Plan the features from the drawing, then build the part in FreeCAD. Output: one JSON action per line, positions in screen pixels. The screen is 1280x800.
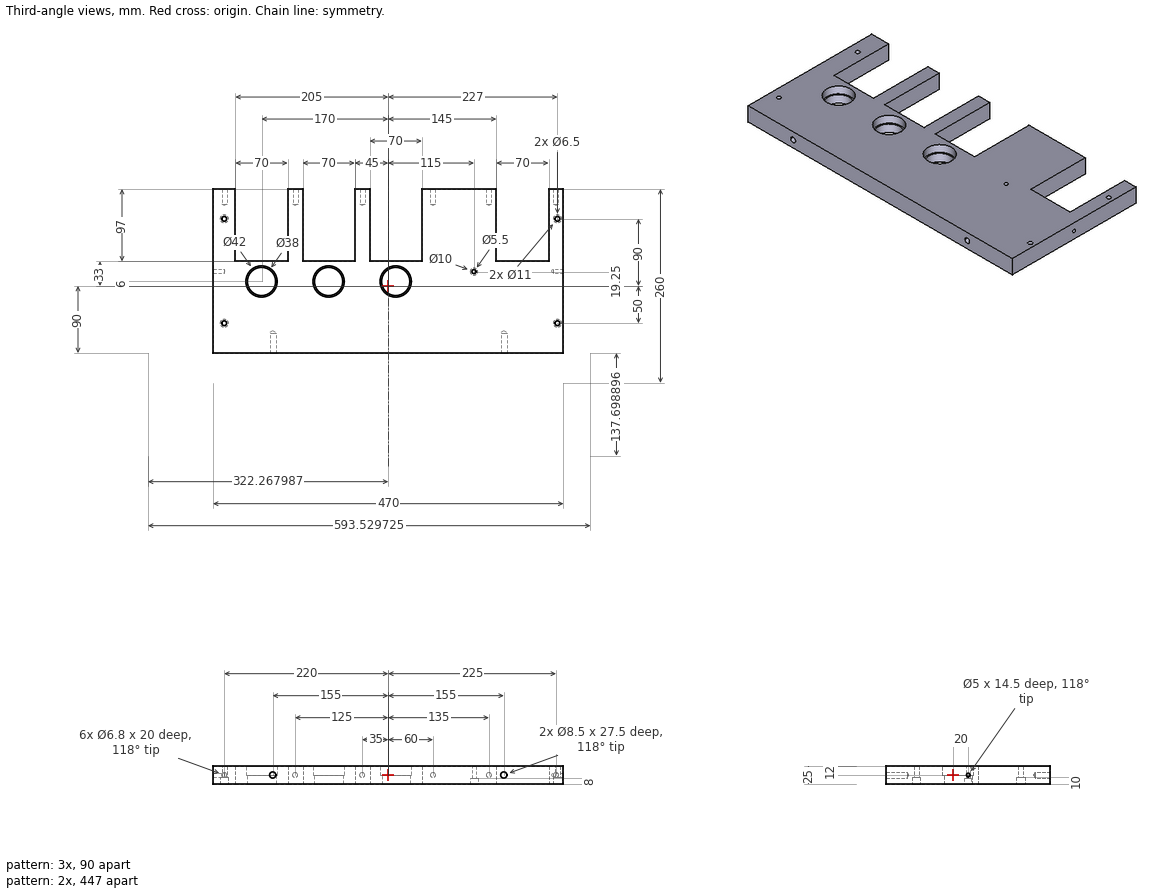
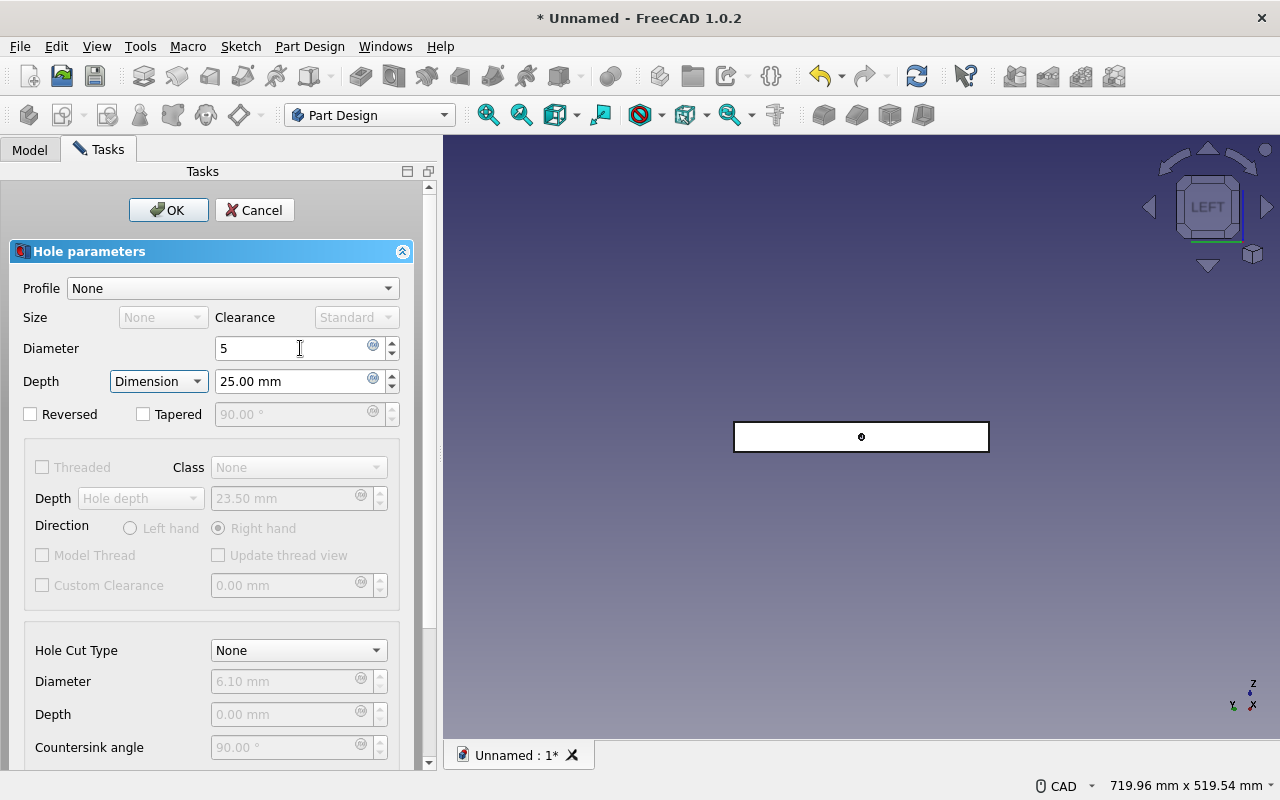
{"action": "triple_click", "coordinate": [300, 382]}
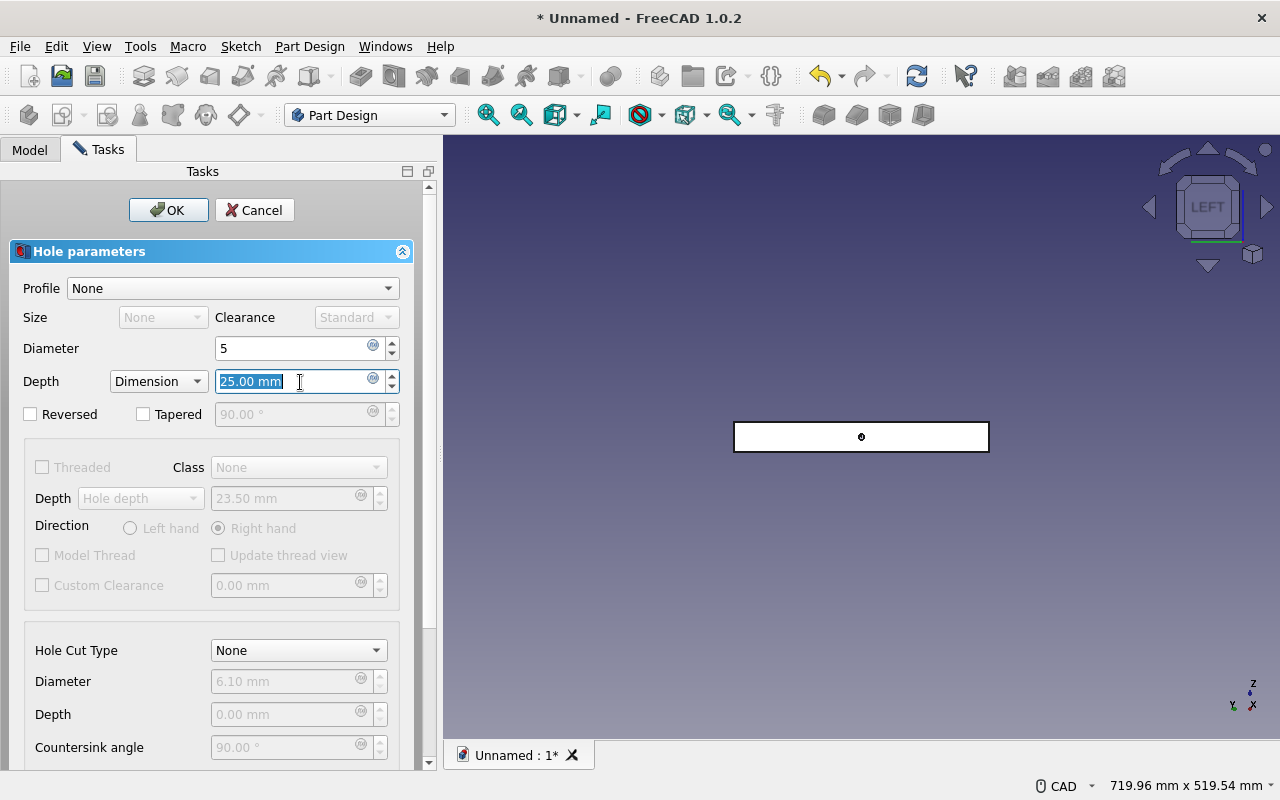
{"action": "type", "text": "14.5"}
{"action": "key", "text": "Tab"}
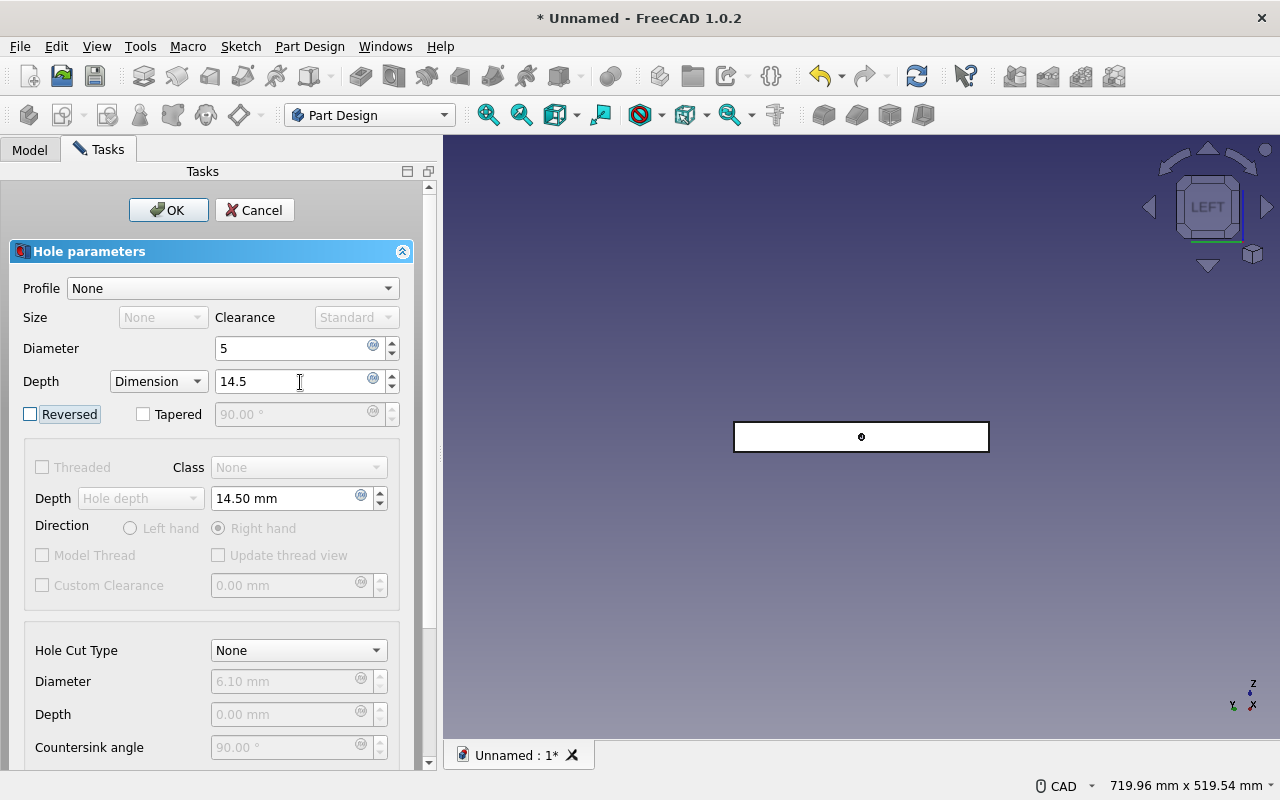
{"action": "left_click", "coordinate": [169, 210]}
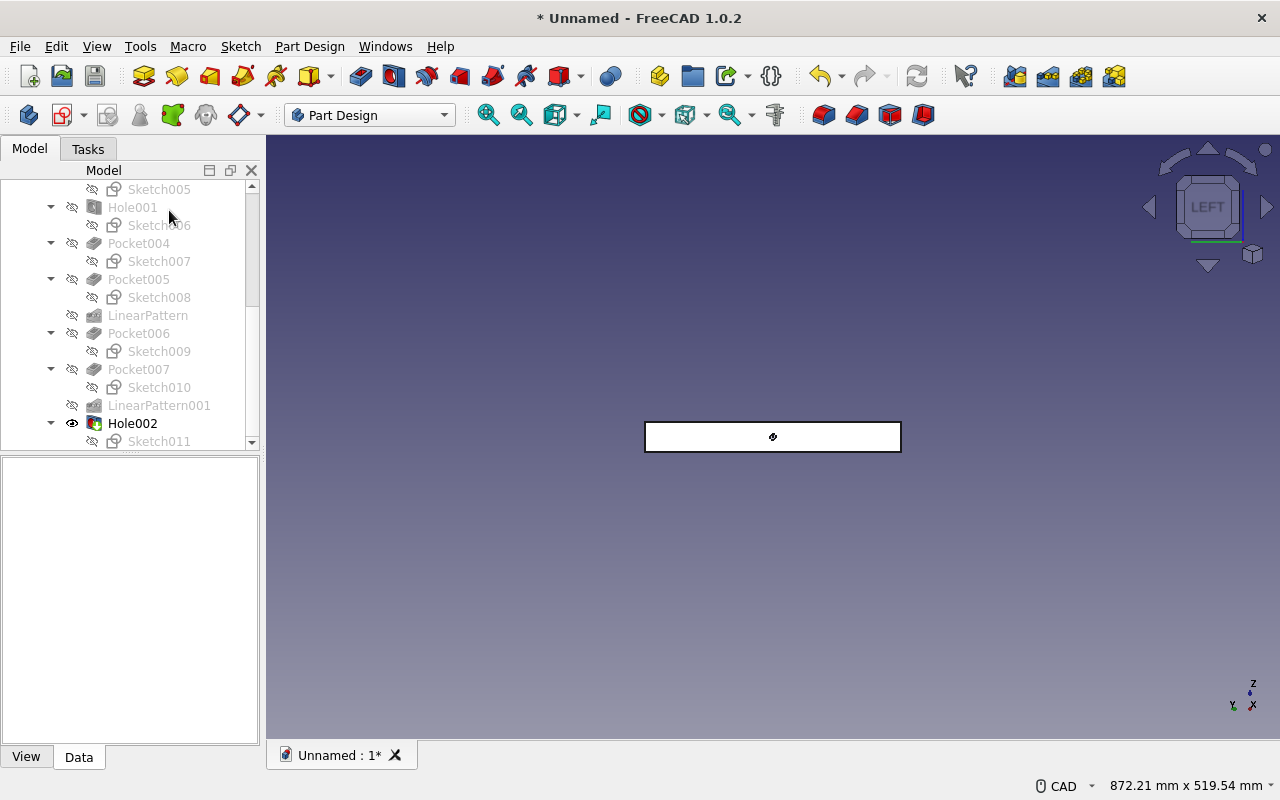
{"action": "left_click", "coordinate": [489, 116]}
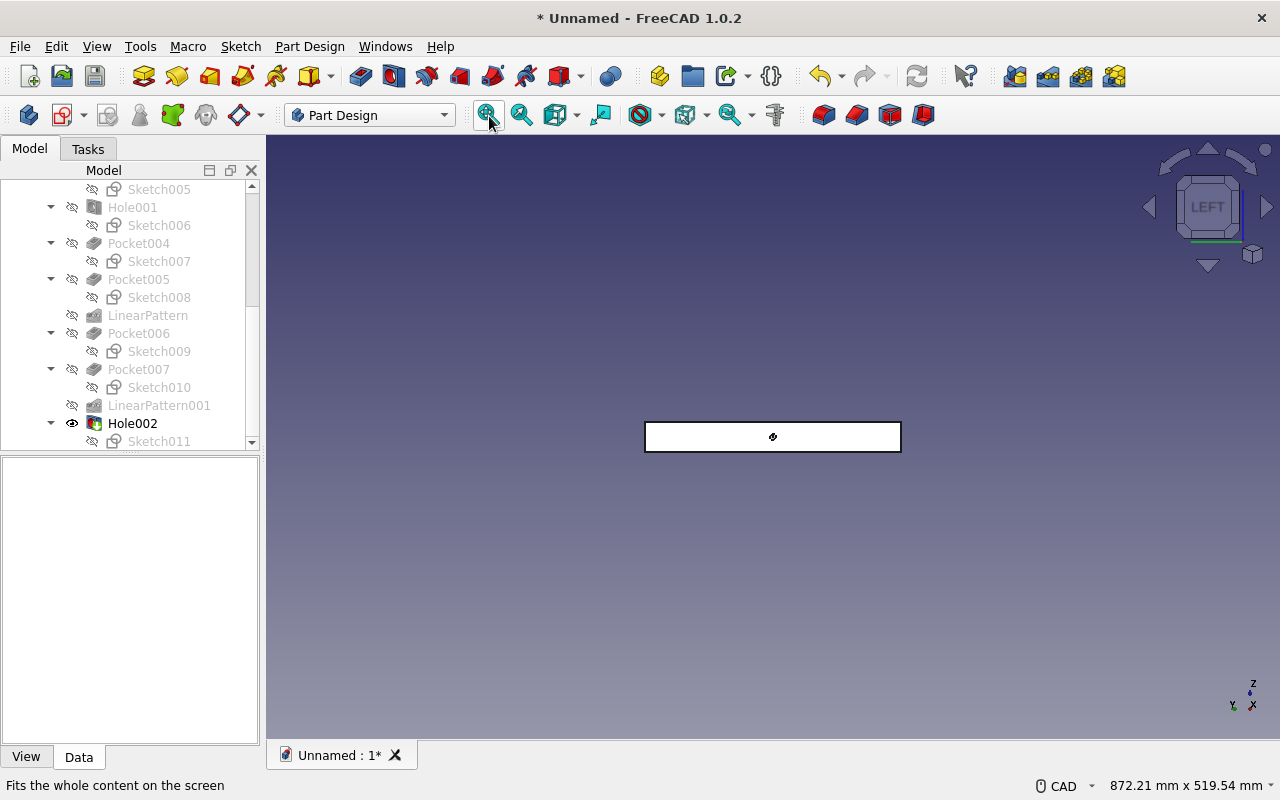
{"action": "key", "text": "0"}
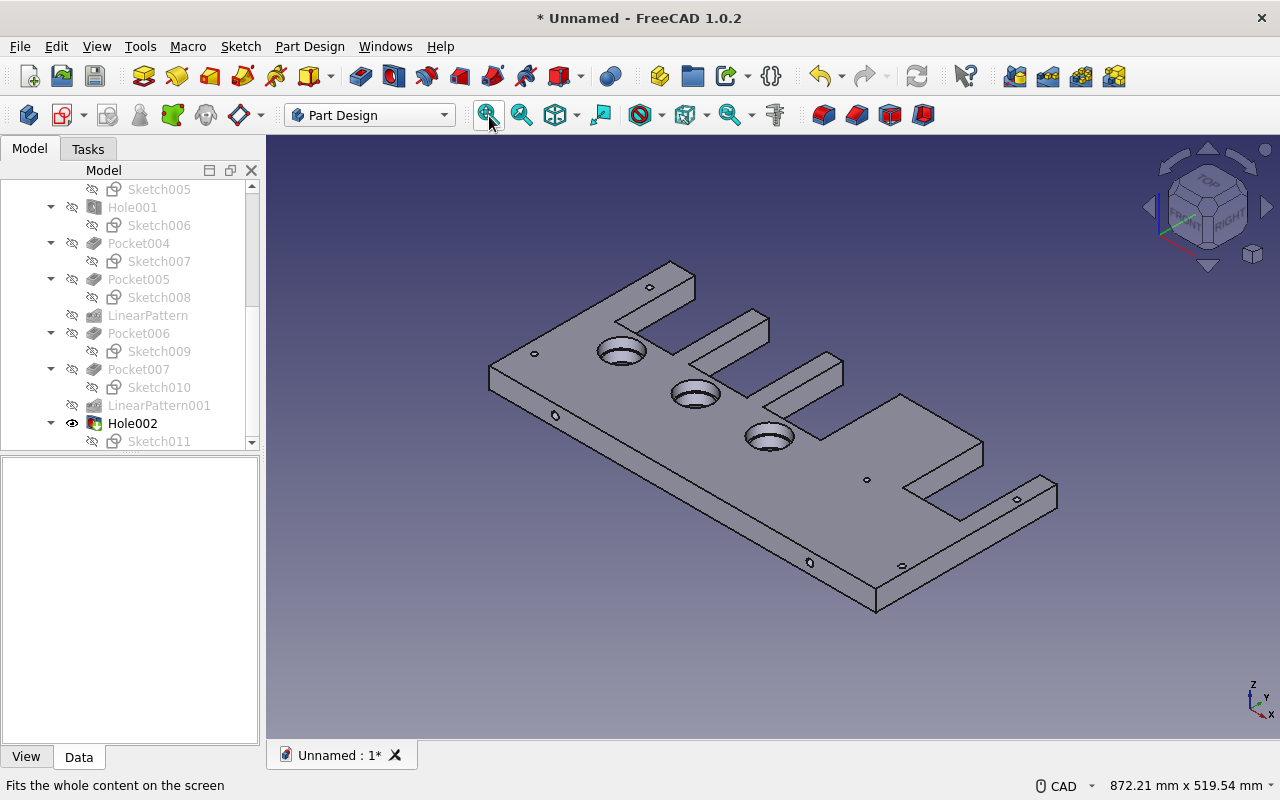
{"action": "left_click", "coordinate": [1044, 503]}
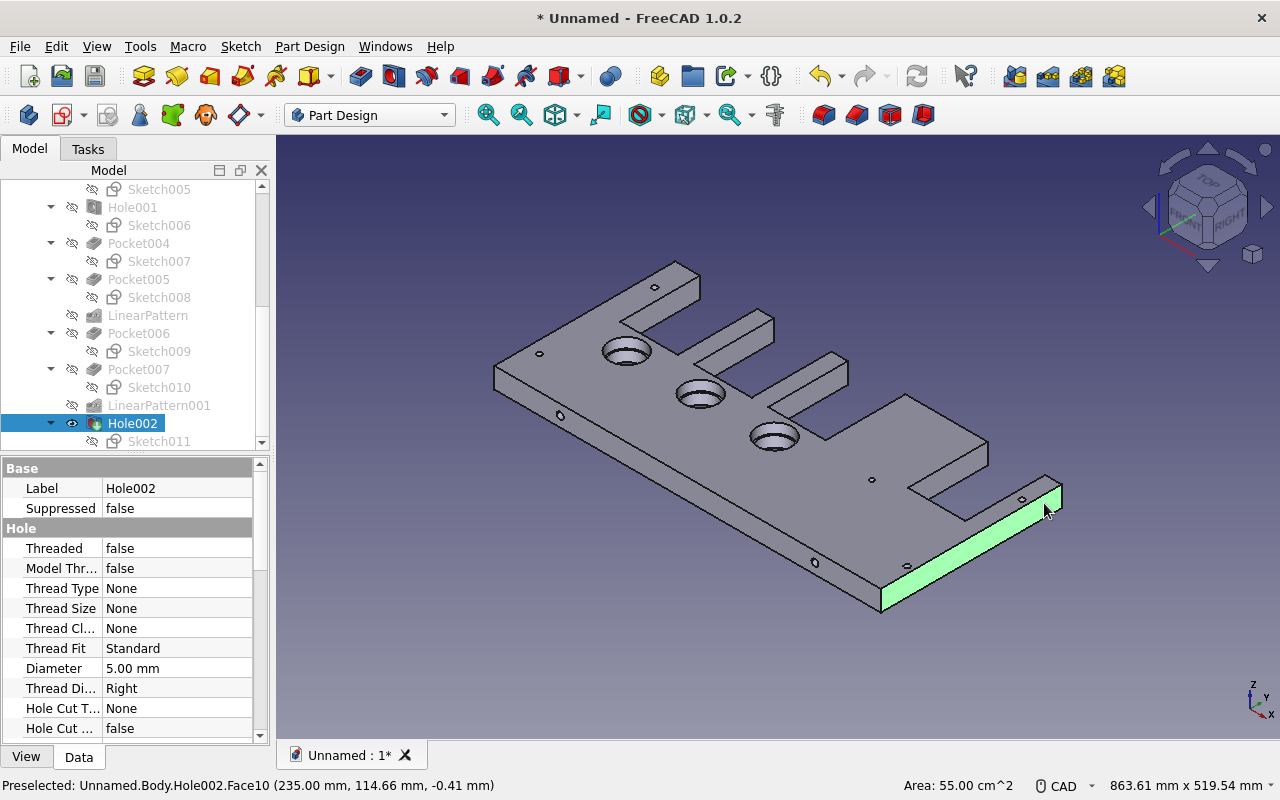
{"action": "left_click", "coordinate": [62, 116]}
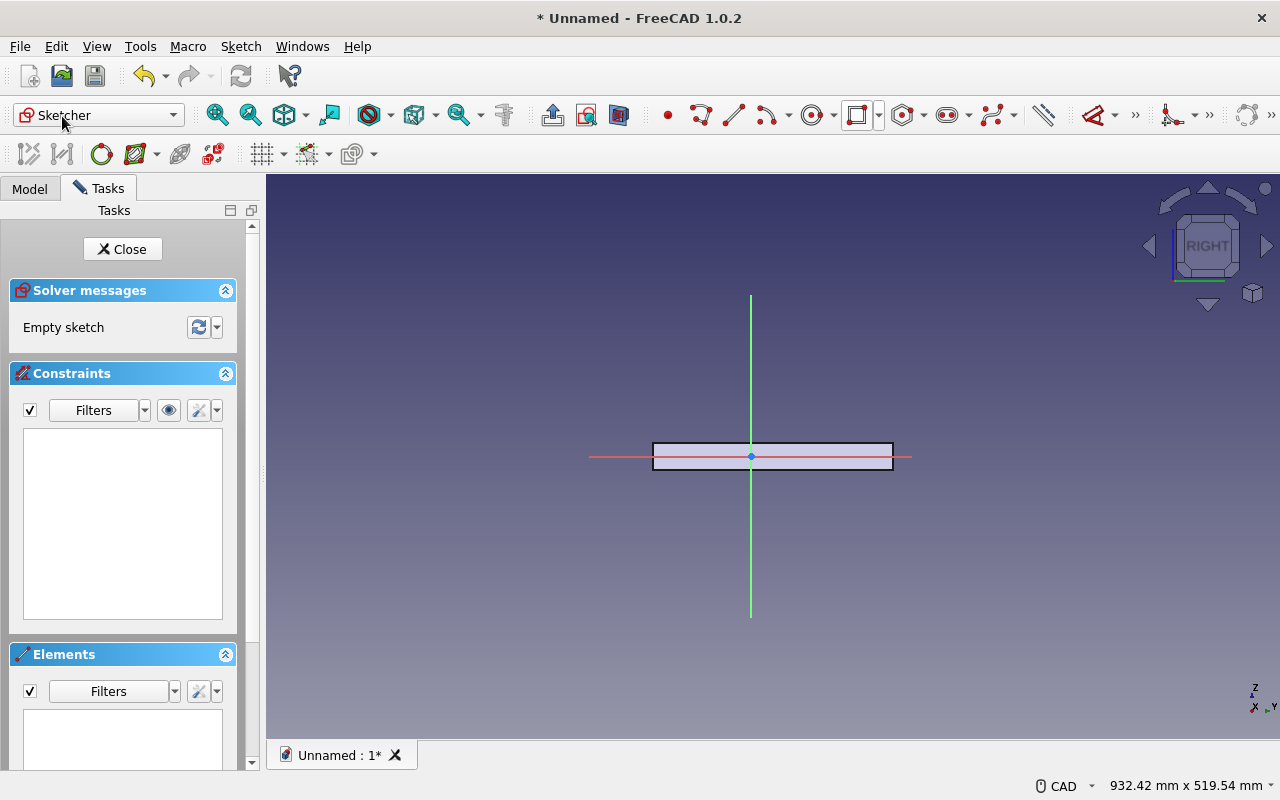
{"action": "scroll", "coordinate": [777, 456], "scroll_direction": "up", "scroll_amount": 15}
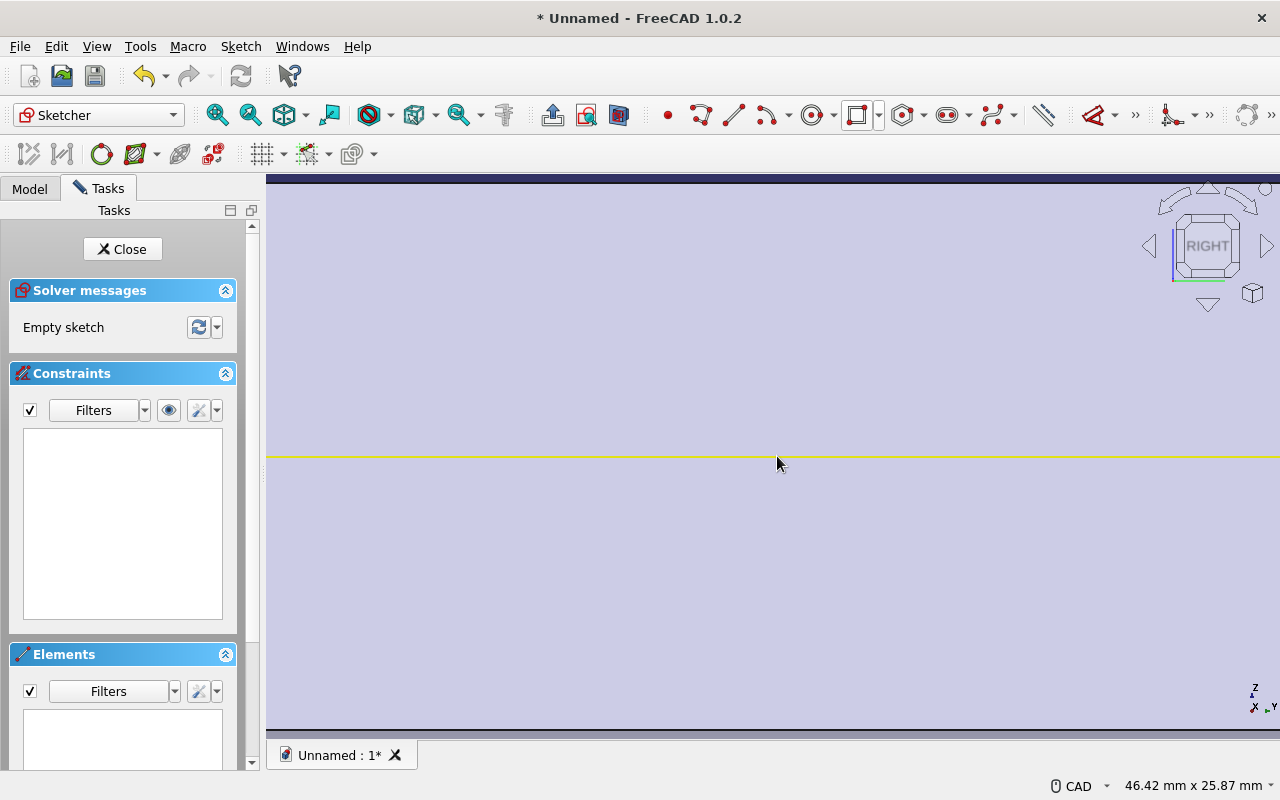
{"action": "scroll", "coordinate": [679, 456], "scroll_direction": "up", "scroll_amount": 6}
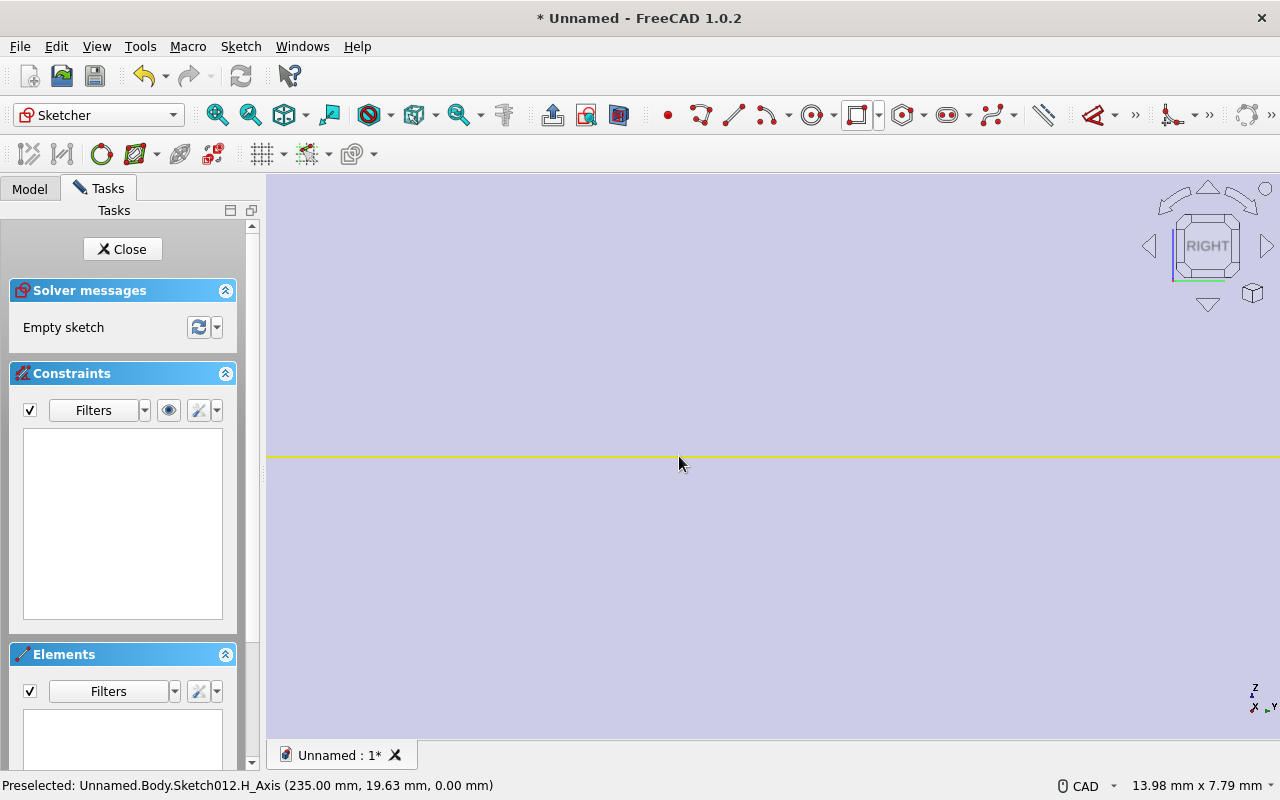
{"action": "left_click", "coordinate": [812, 116]}